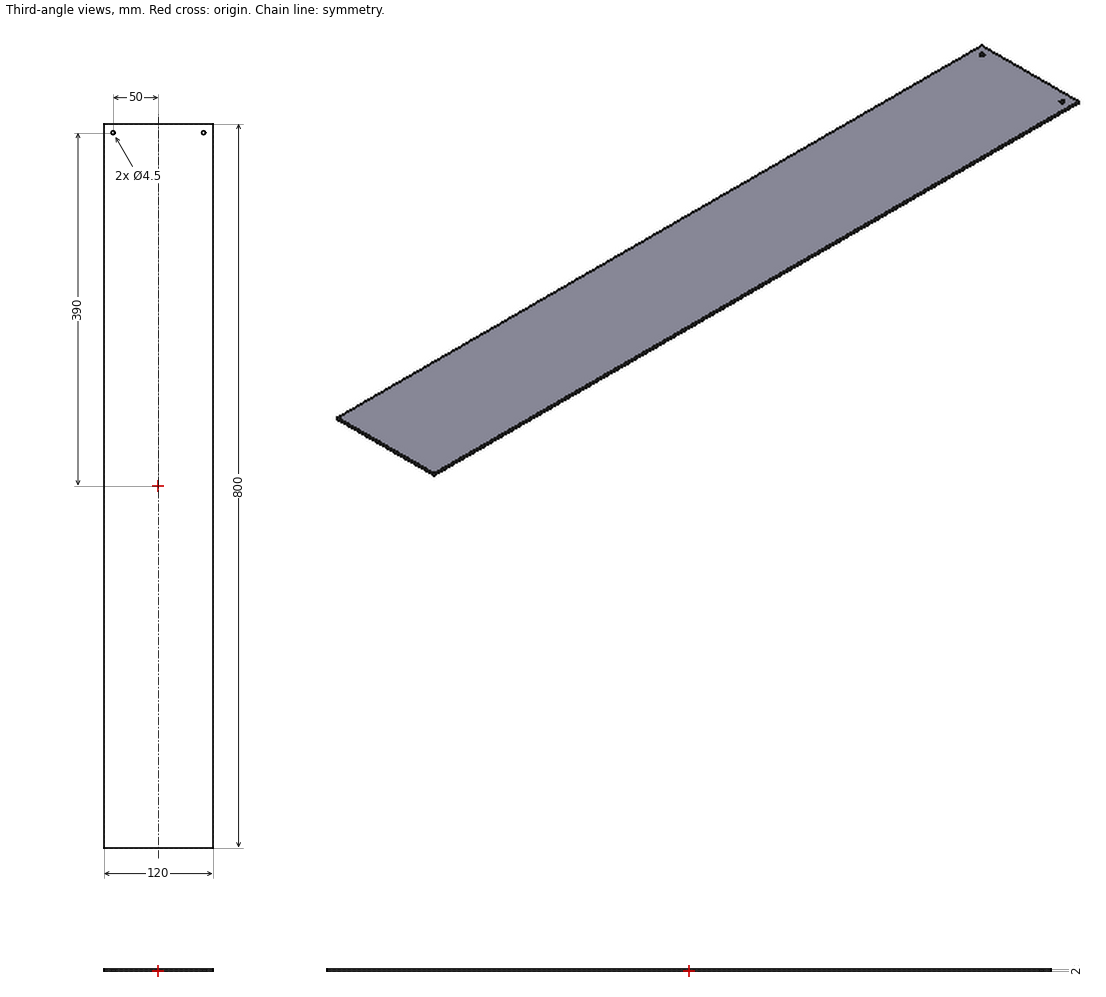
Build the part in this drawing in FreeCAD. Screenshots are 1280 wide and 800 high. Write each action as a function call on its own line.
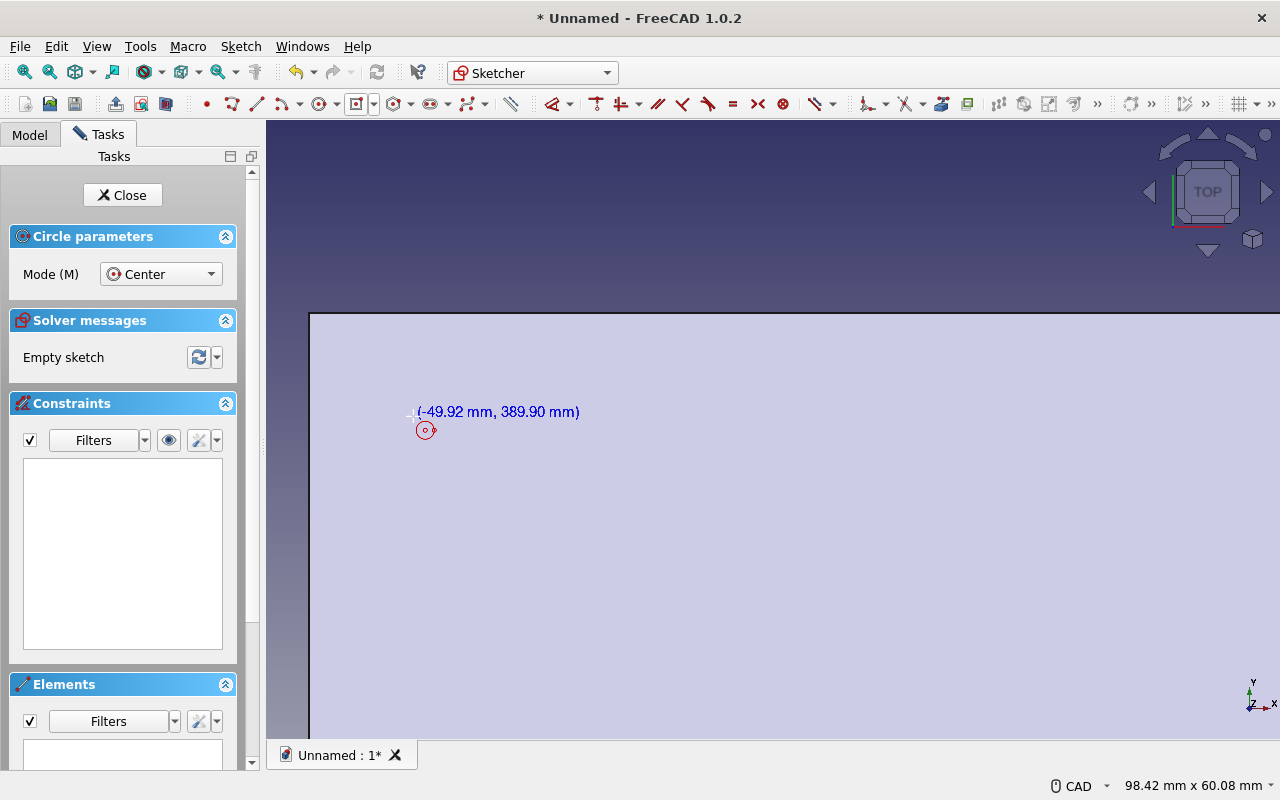
click(412, 416)
move(428, 400)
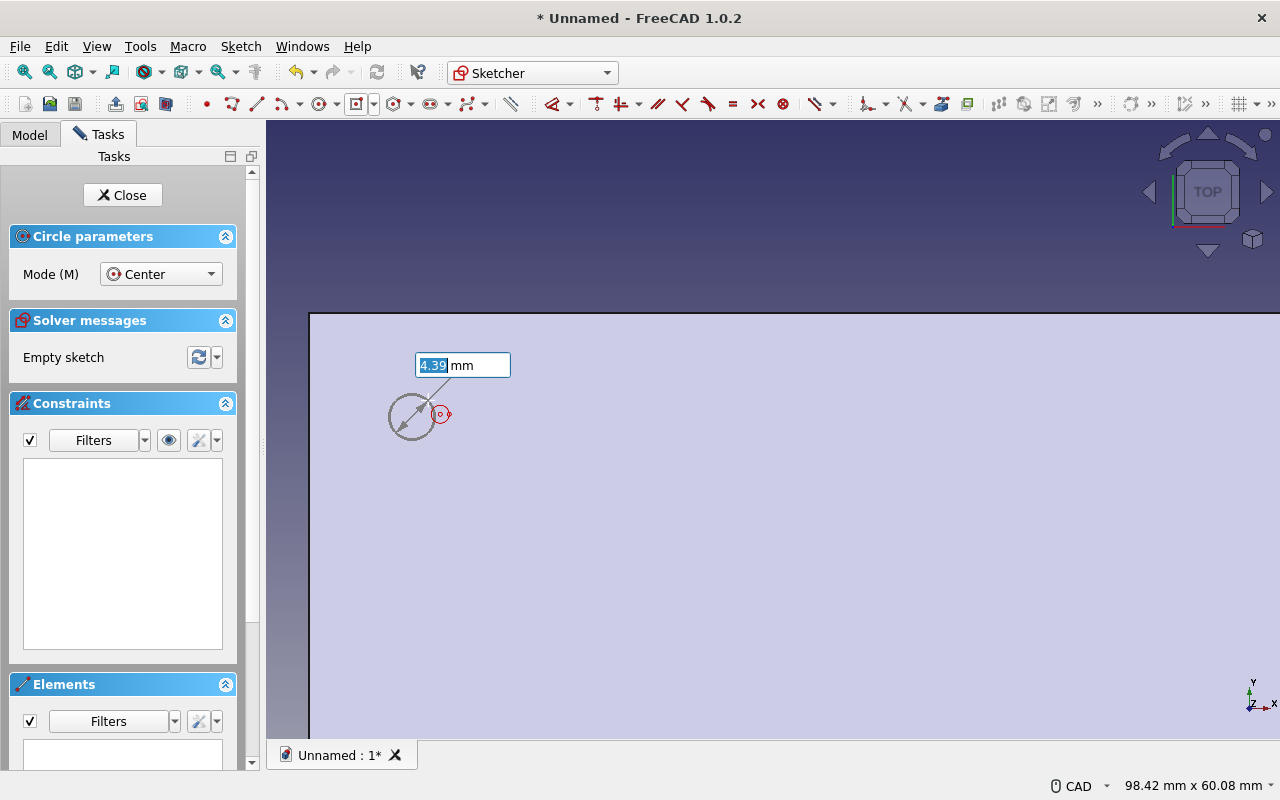
text(4.5)
key(Return)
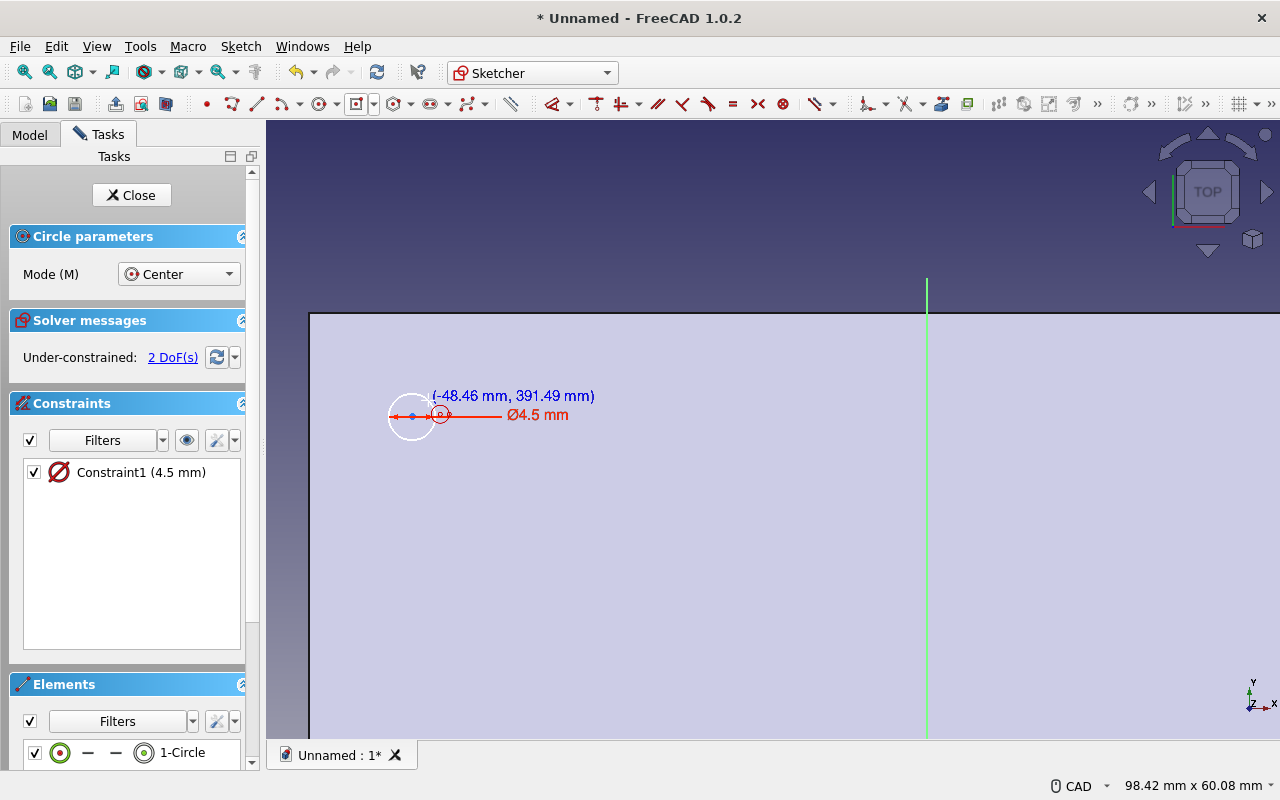
scroll(434, 445, down, 3)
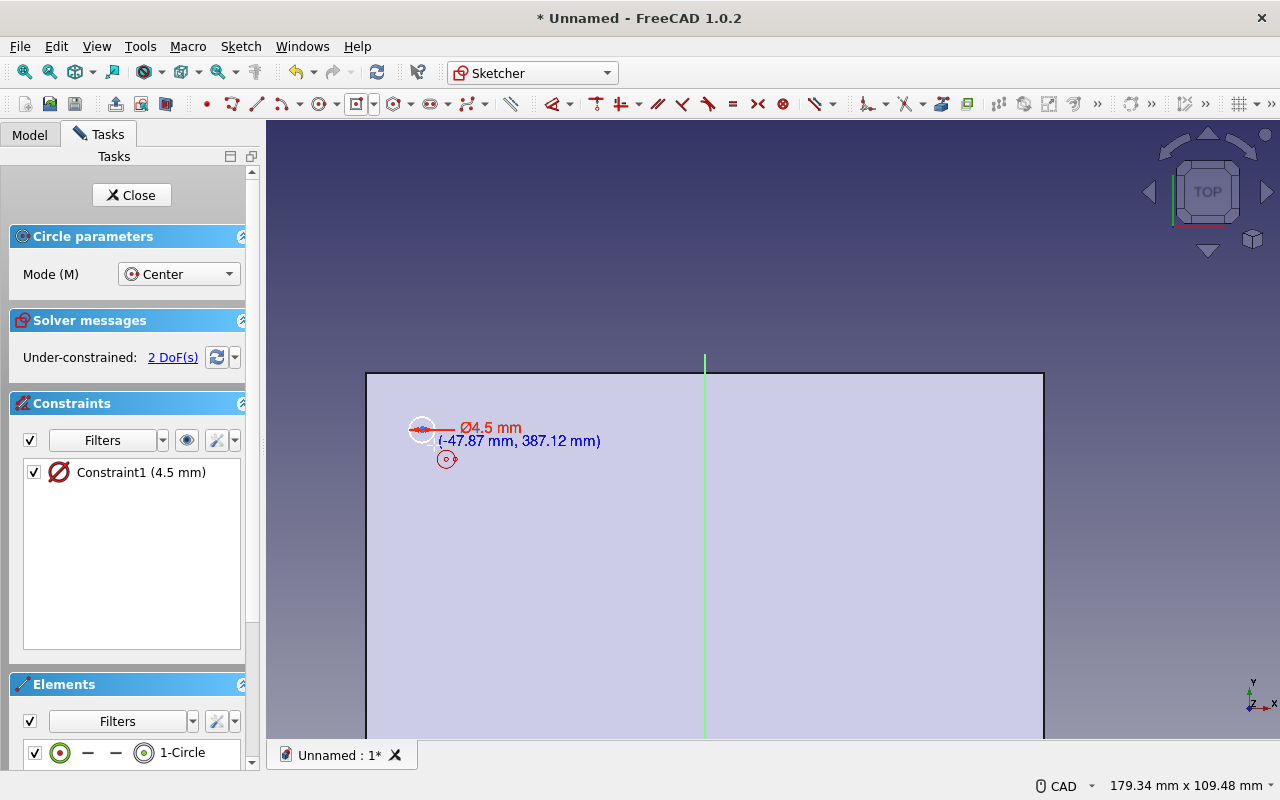
scroll(987, 430, up, 3)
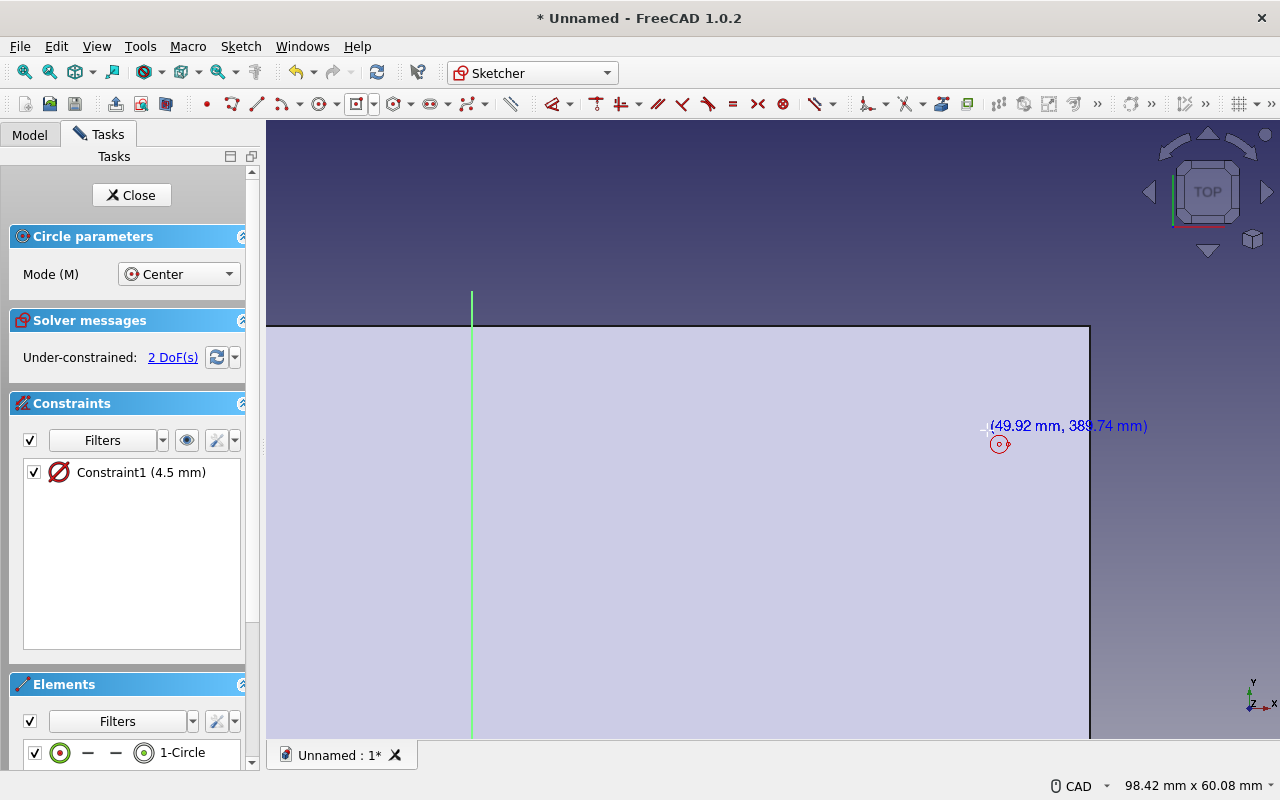
click(987, 429)
move(1004, 412)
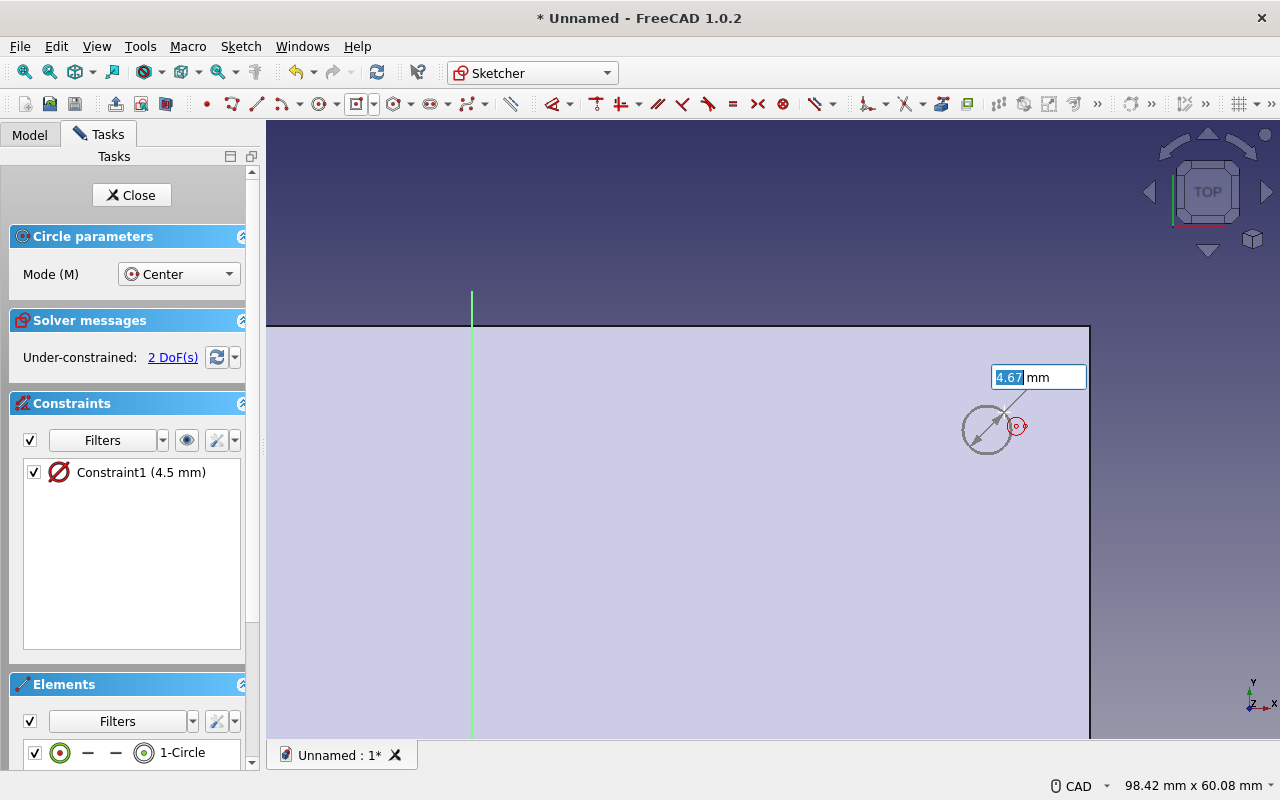
text(4.5)
key(Return)
key(Escape)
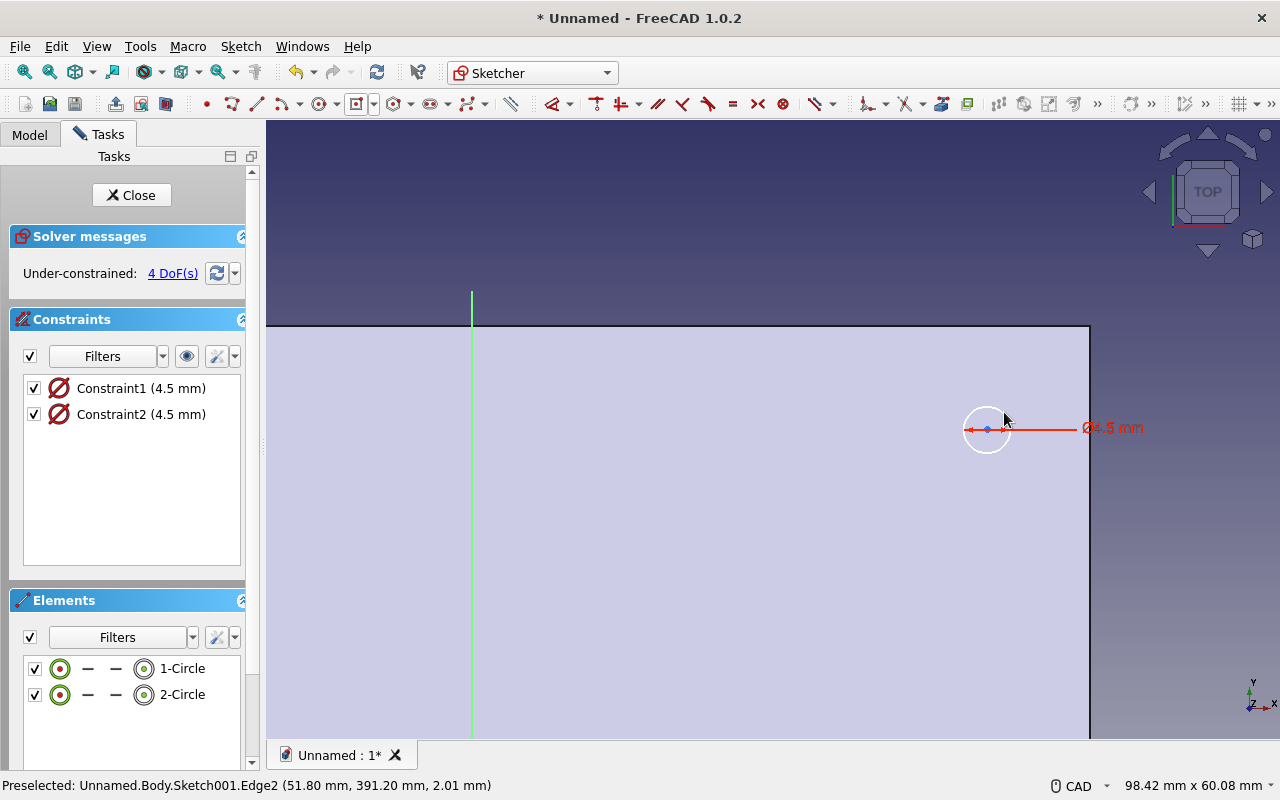
scroll(987, 430, down, 3)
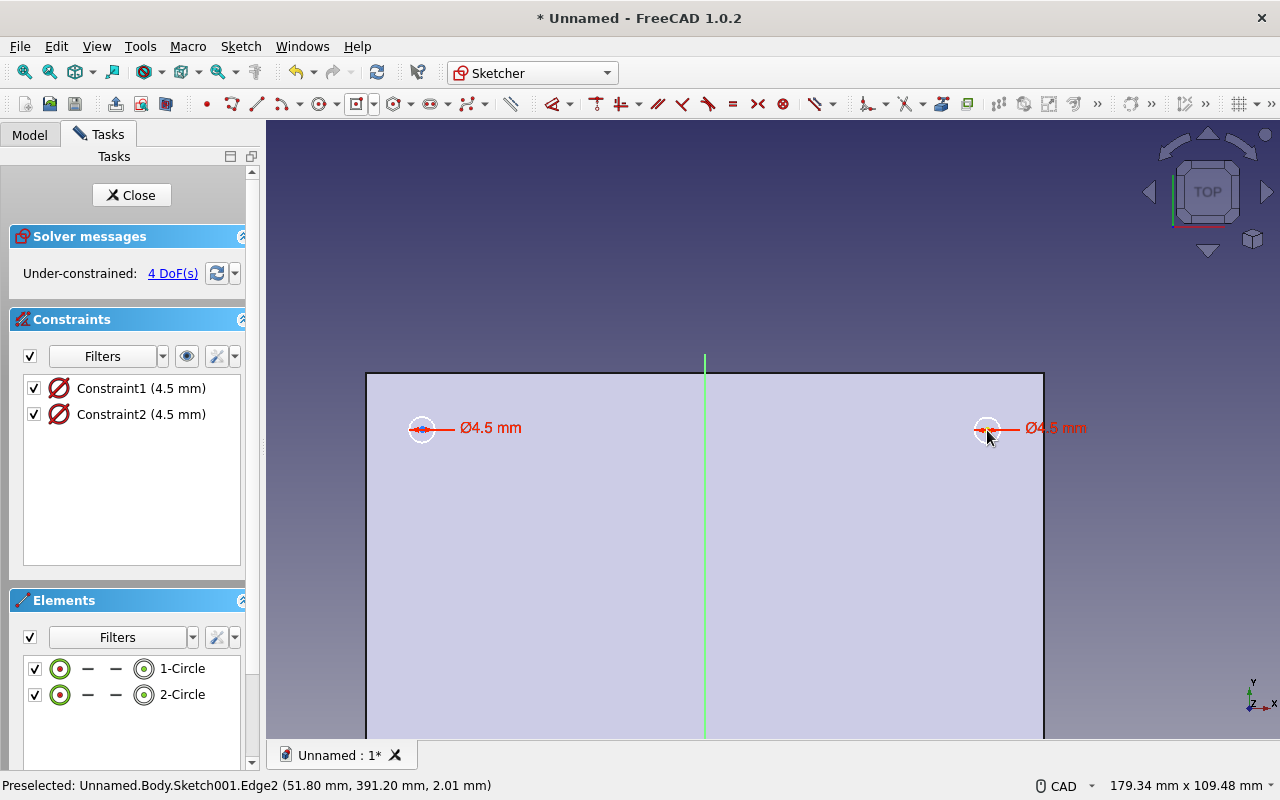
click(422, 430)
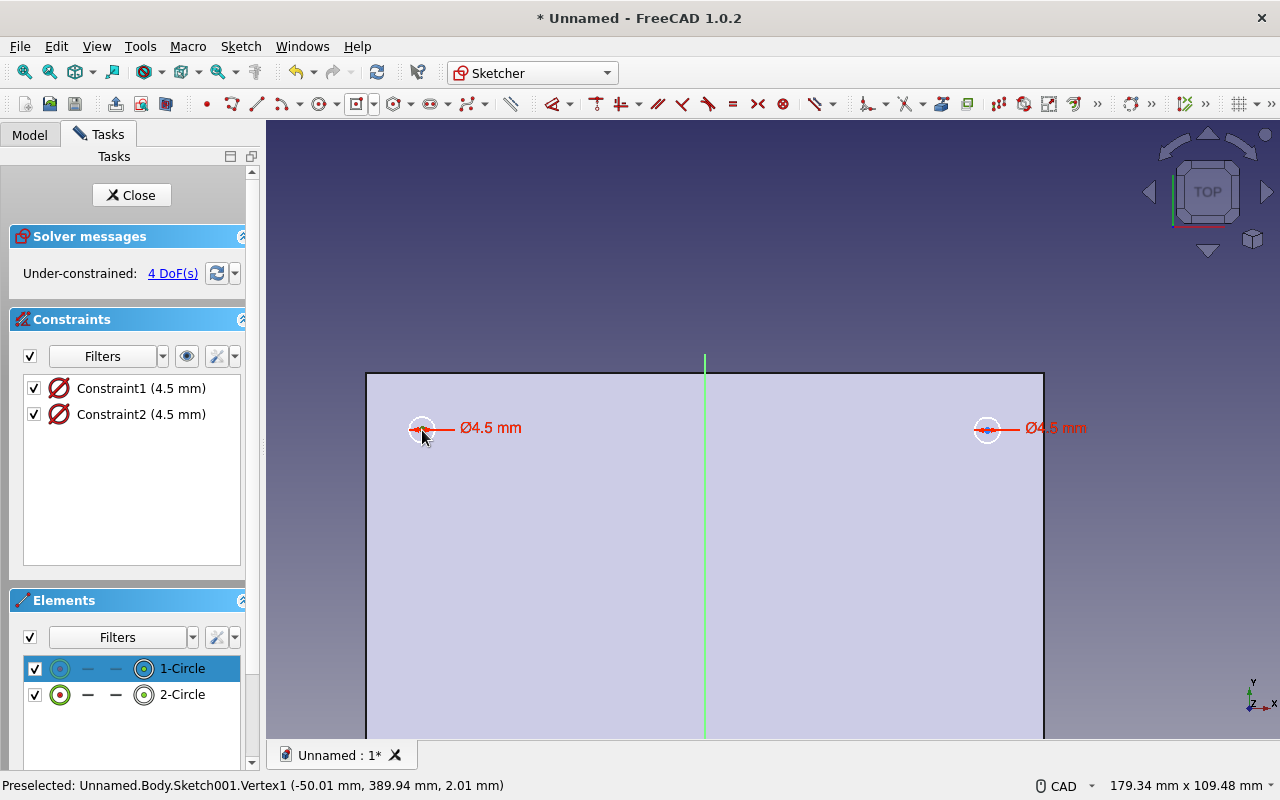
click(987, 430)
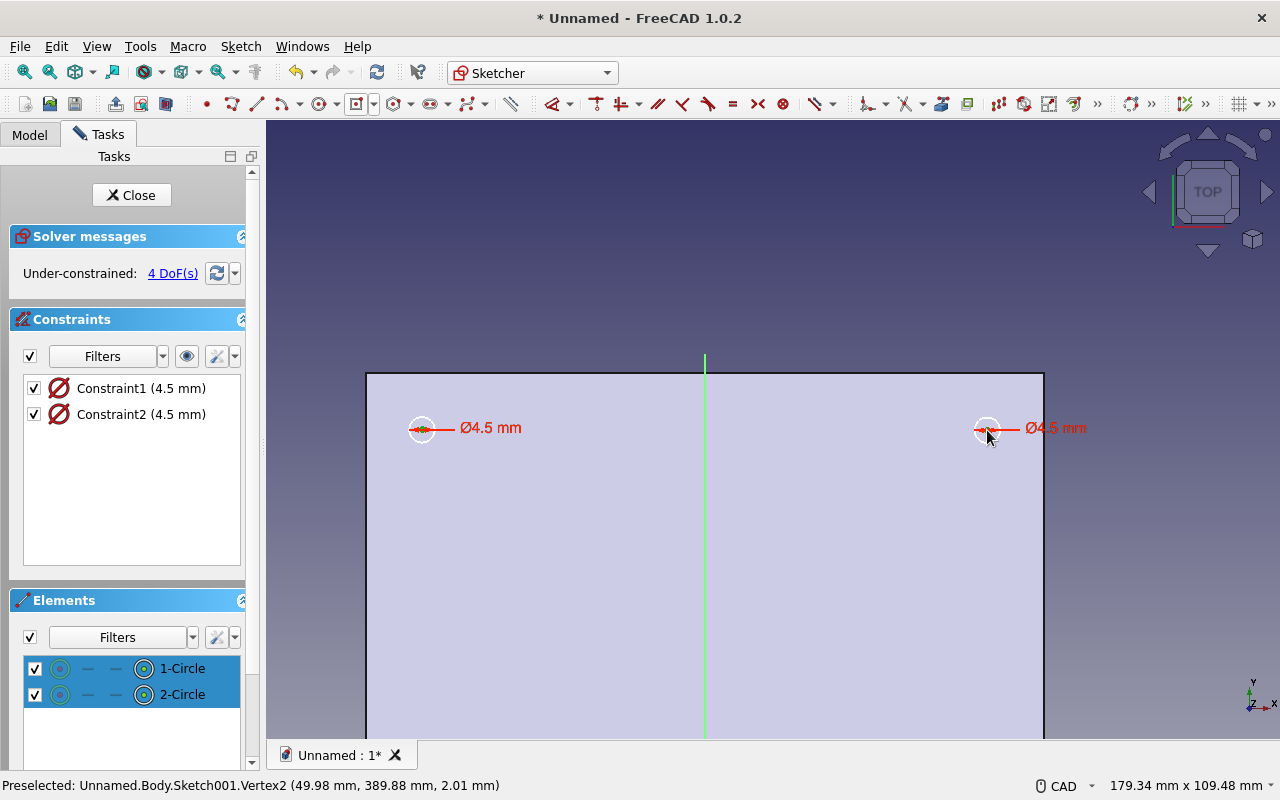
click(705, 671)